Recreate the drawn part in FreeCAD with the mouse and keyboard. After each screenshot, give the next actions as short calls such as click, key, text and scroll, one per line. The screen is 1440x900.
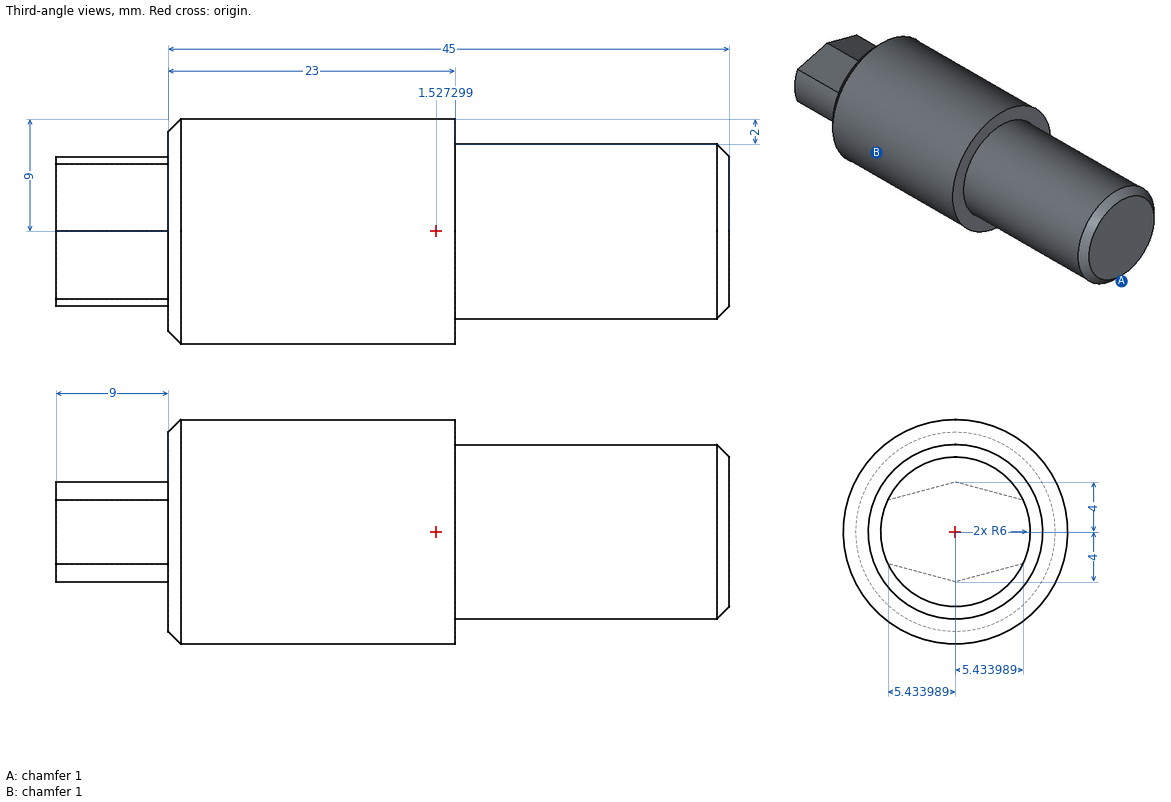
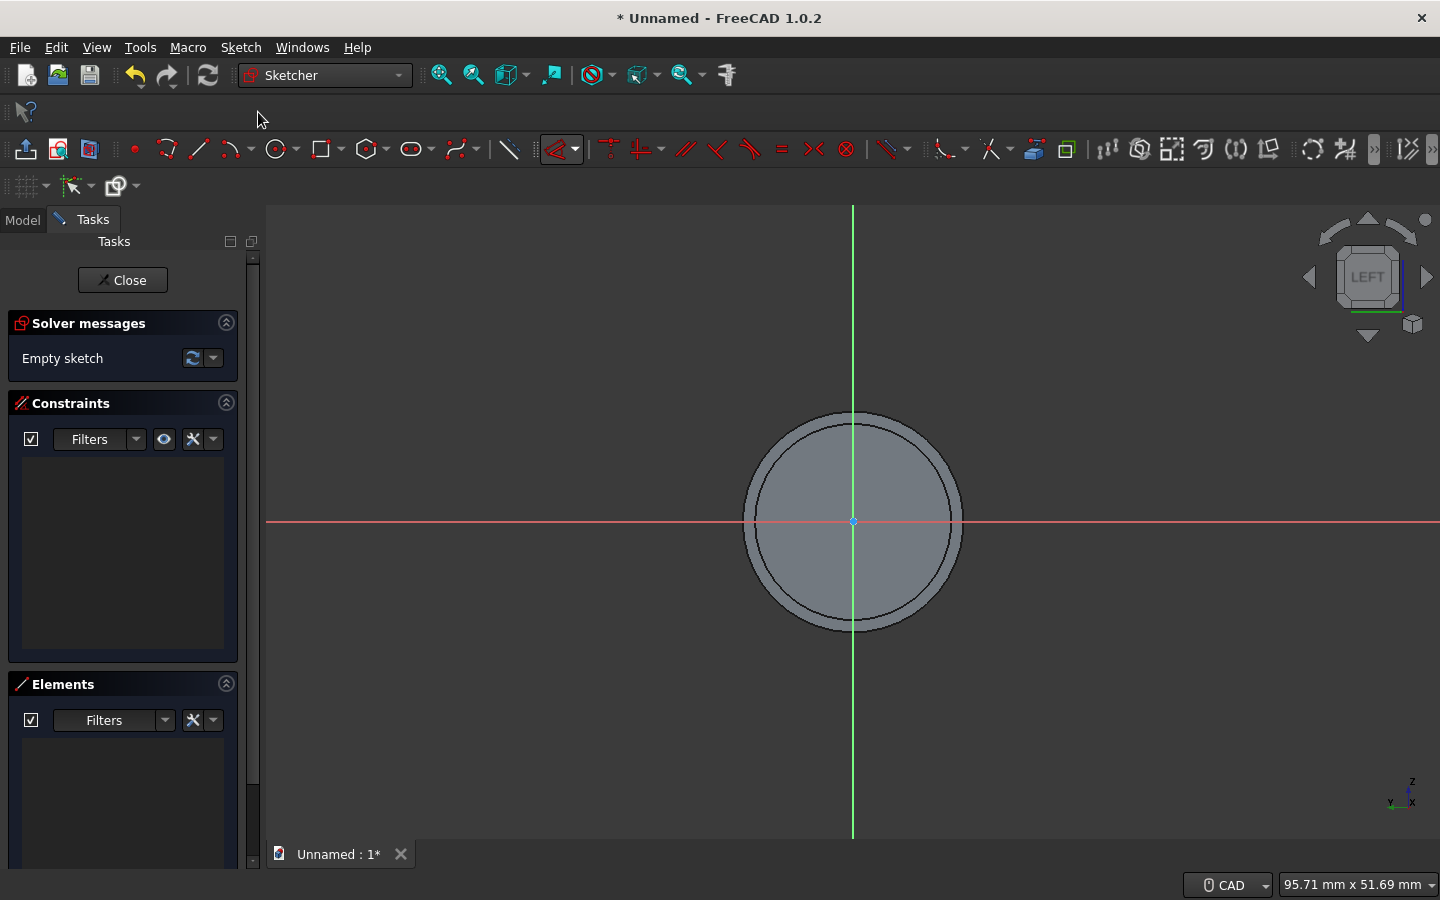
scroll(876, 522, up, 7)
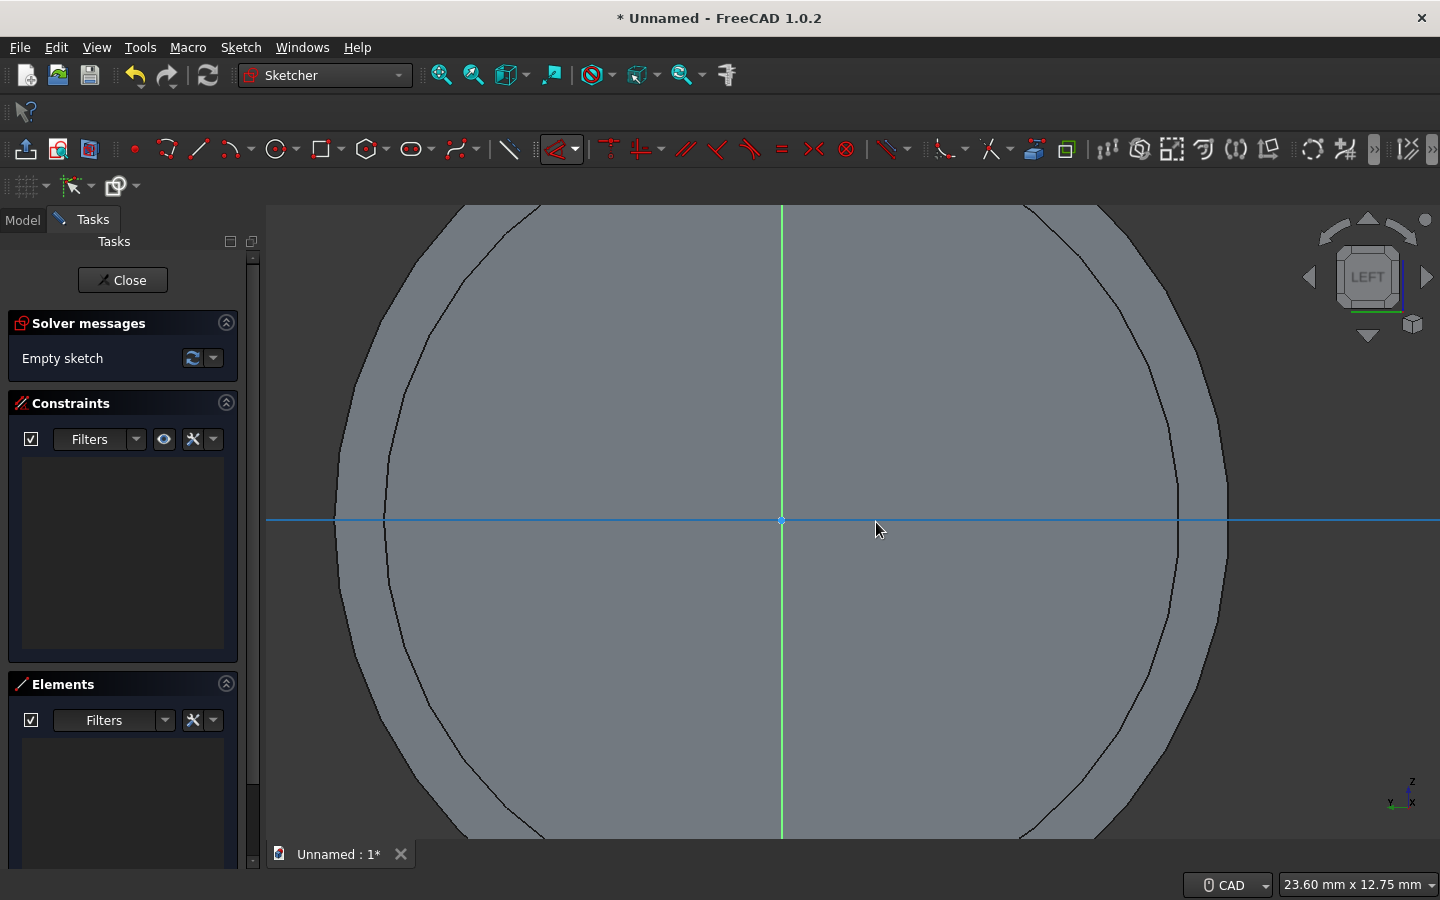
click(168, 150)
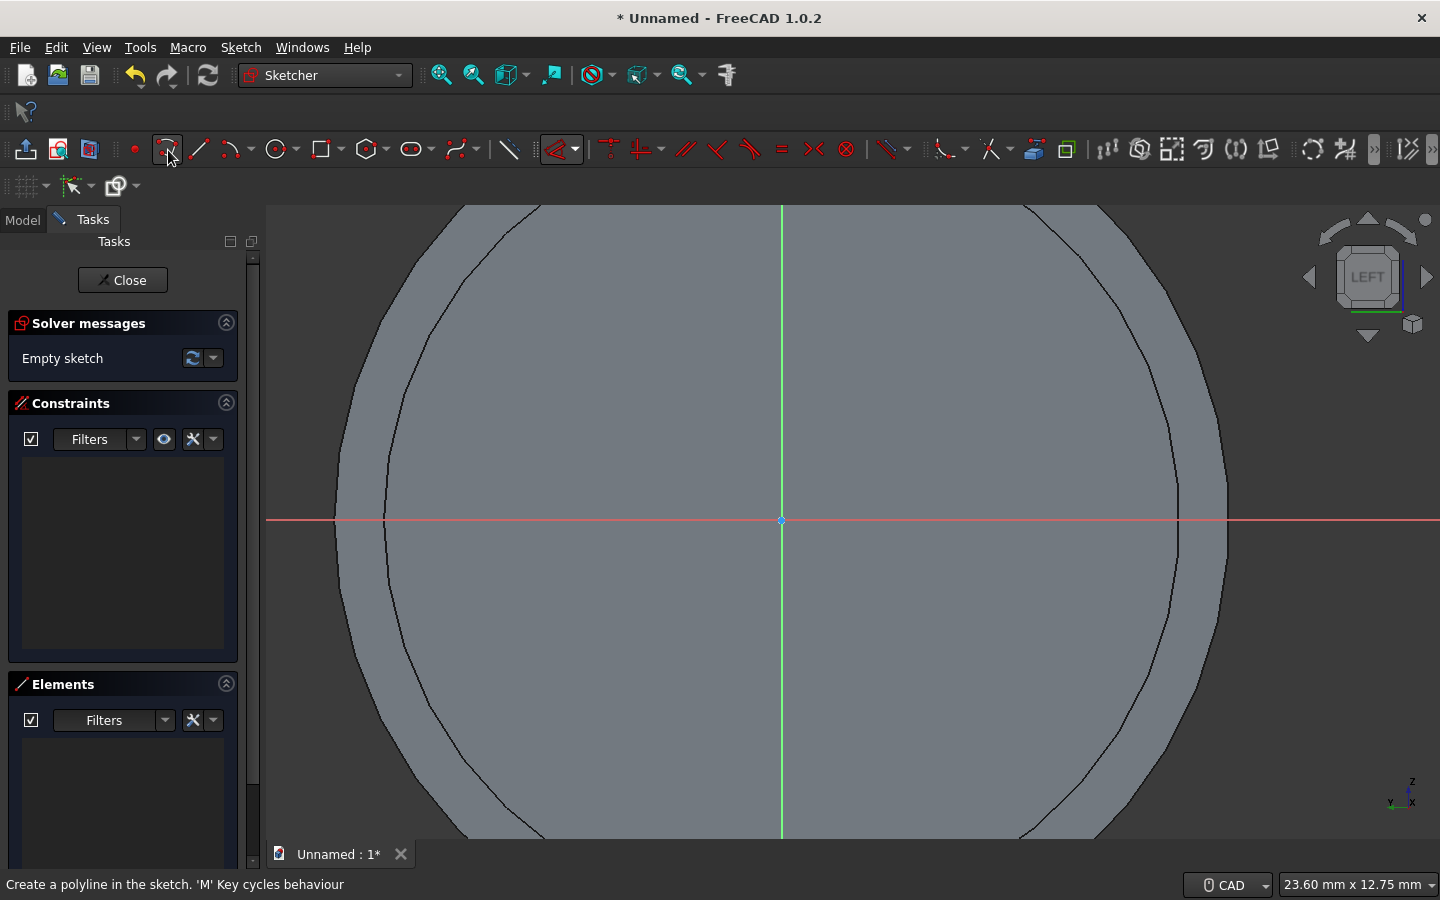
click(512, 647)
click(782, 719)
click(1052, 647)
right_click(1052, 647)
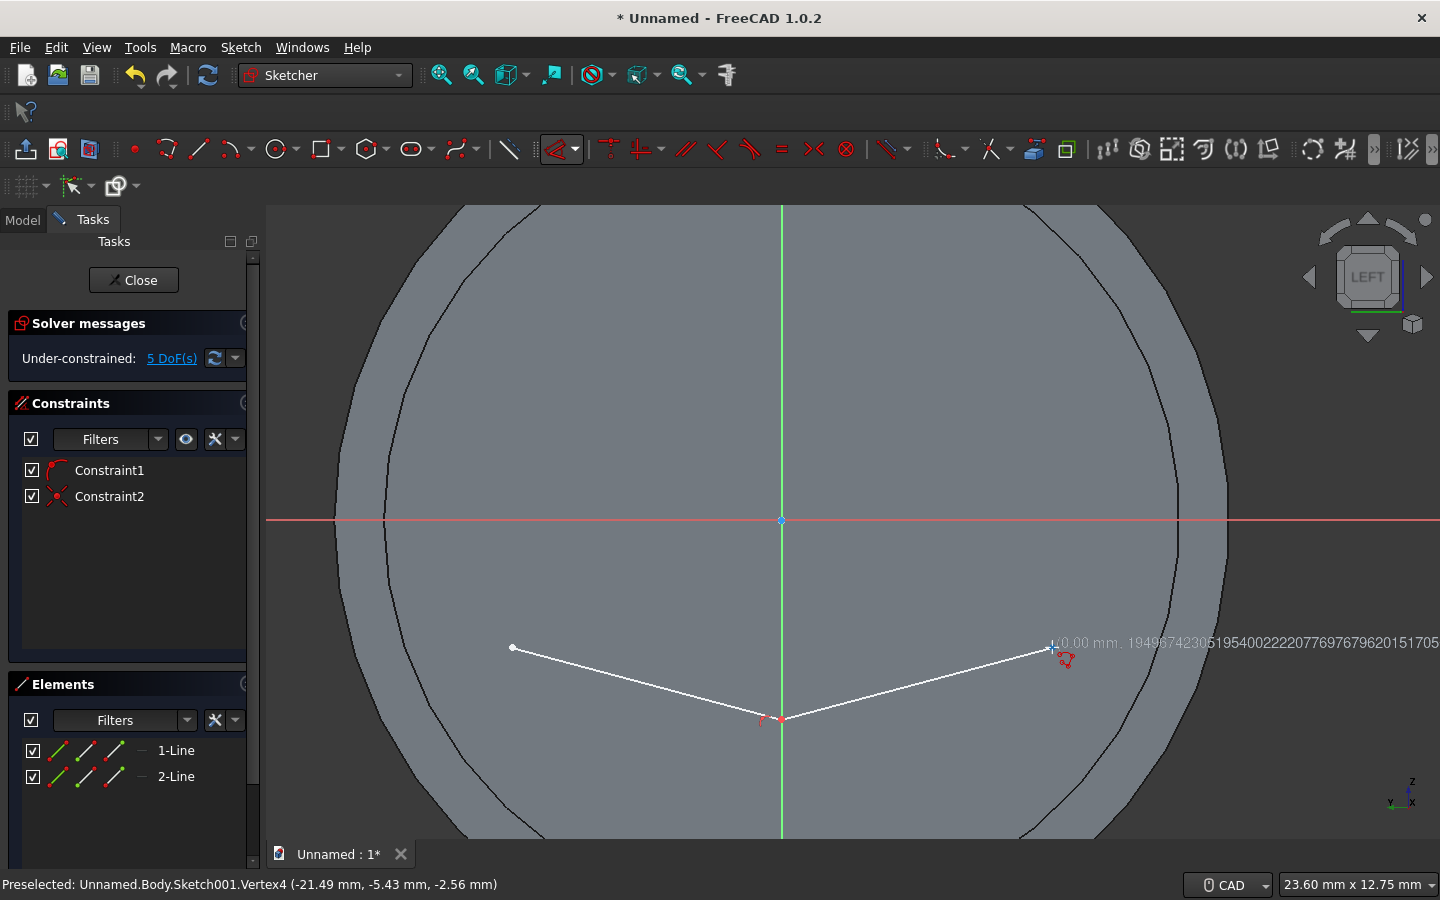
click(1052, 394)
click(782, 322)
click(512, 394)
right_click(512, 394)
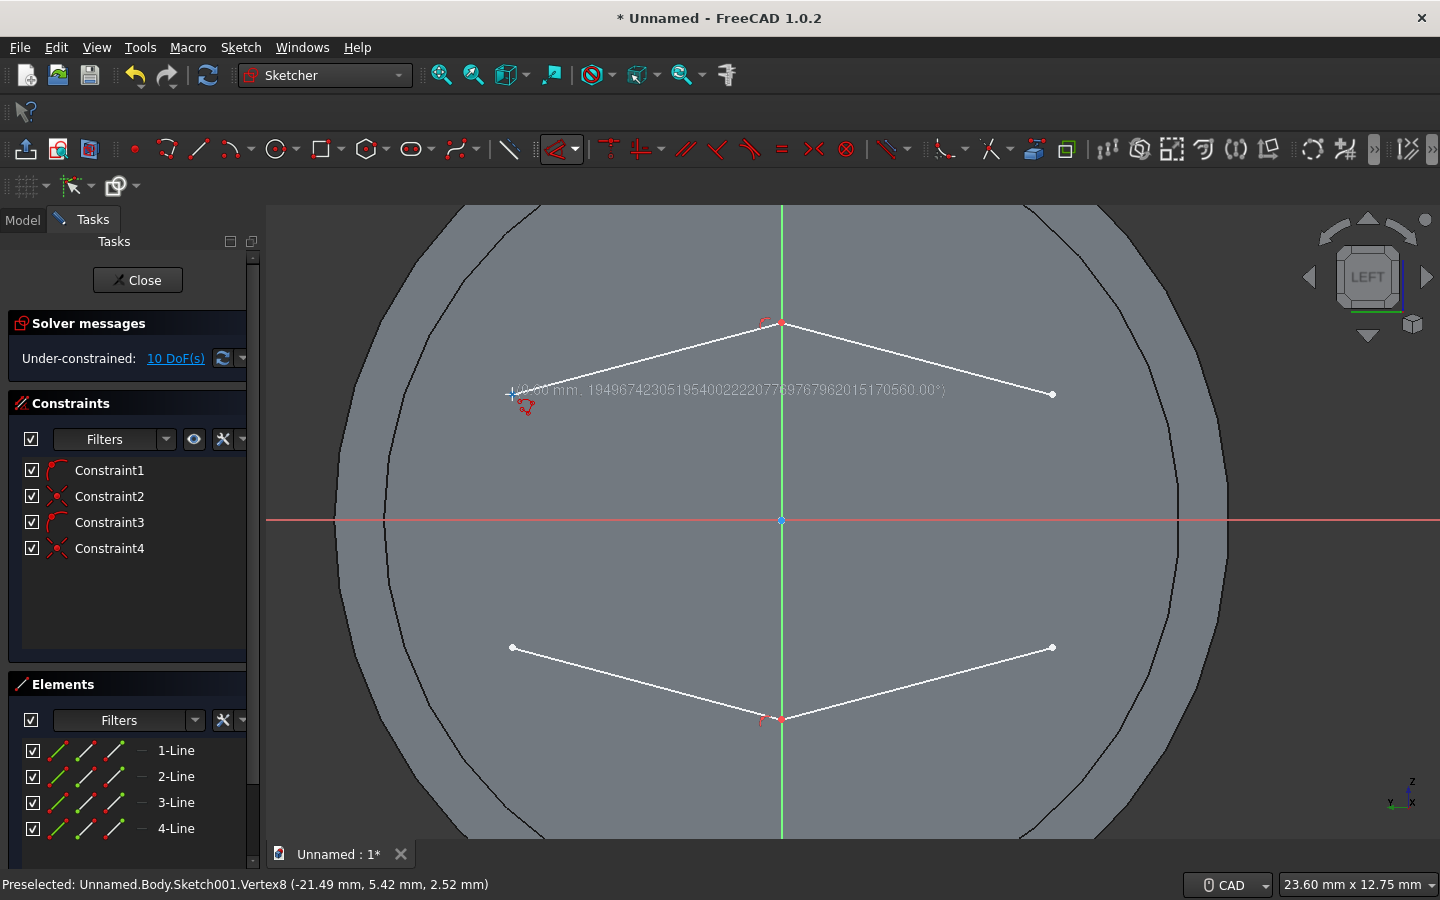
key(g)
key(3)
key(a)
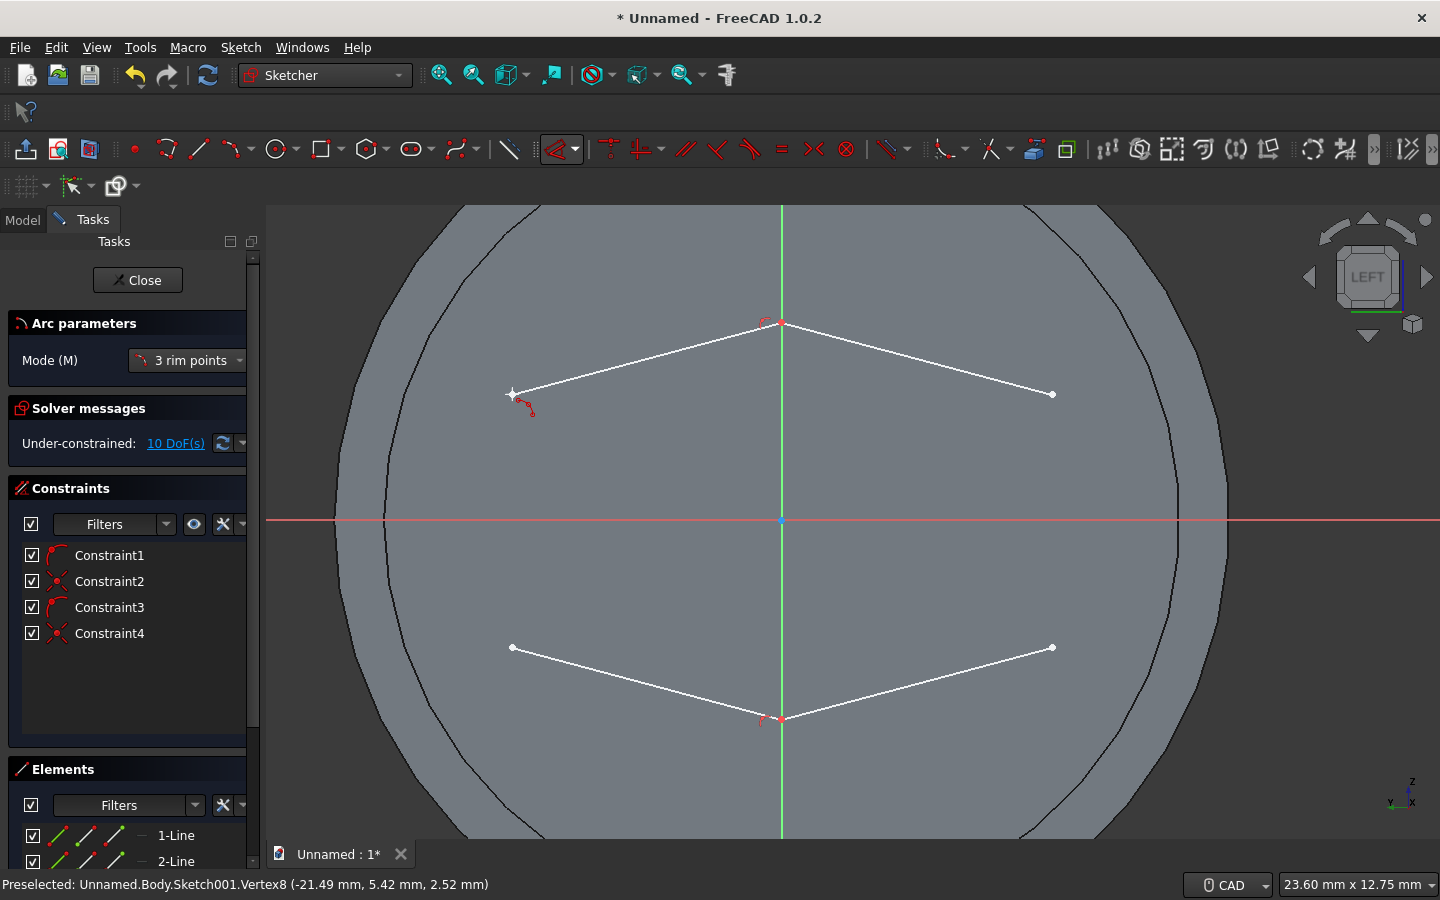
click(1052, 648)
click(1052, 395)
click(1079, 547)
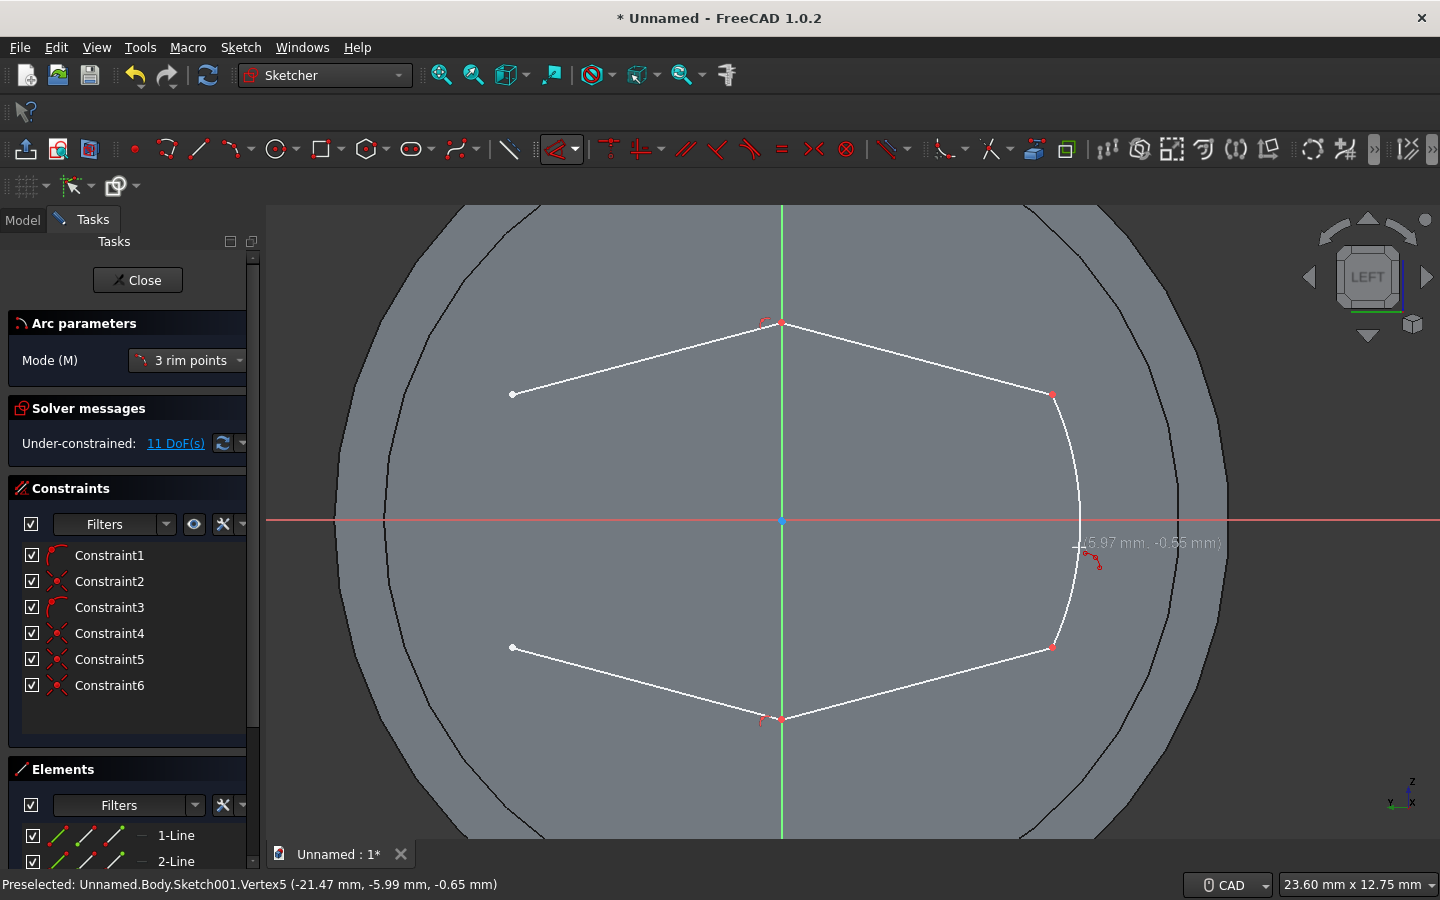
click(512, 395)
click(512, 648)
click(484, 494)
key(Escape)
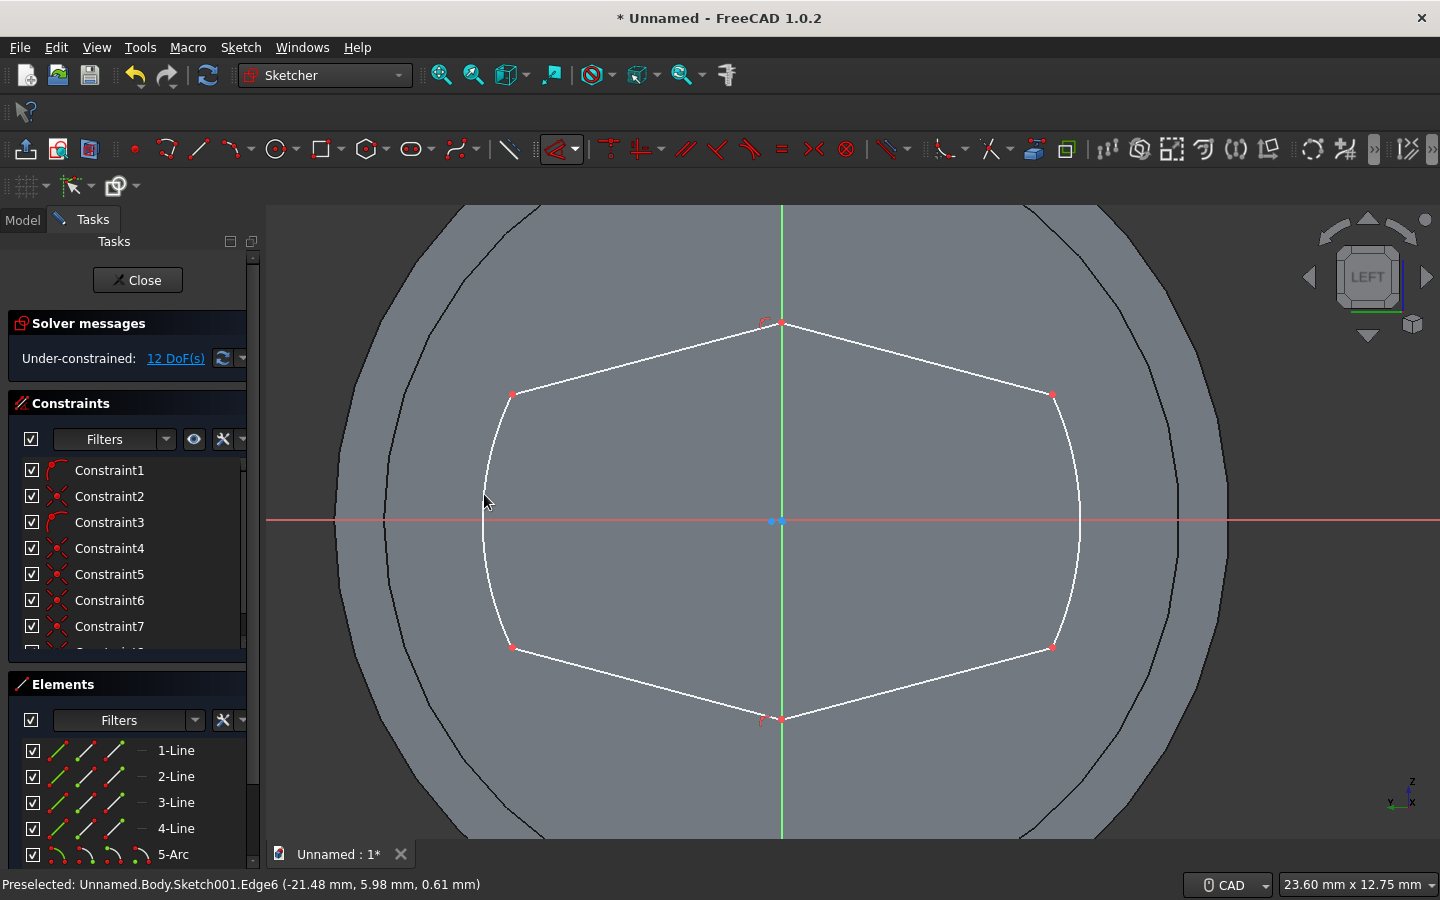
click(1076, 573)